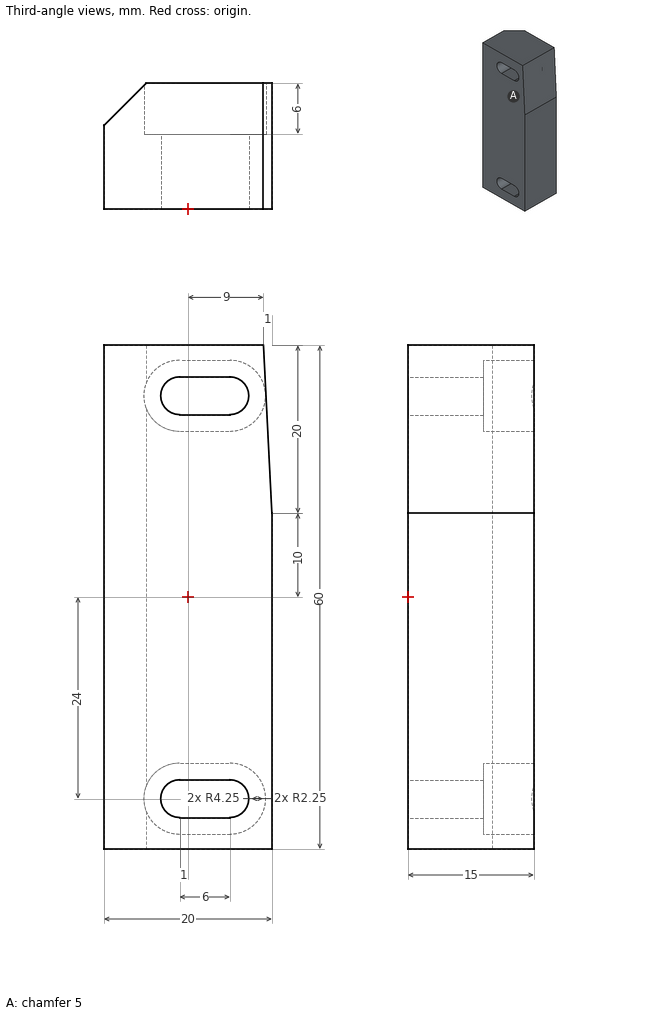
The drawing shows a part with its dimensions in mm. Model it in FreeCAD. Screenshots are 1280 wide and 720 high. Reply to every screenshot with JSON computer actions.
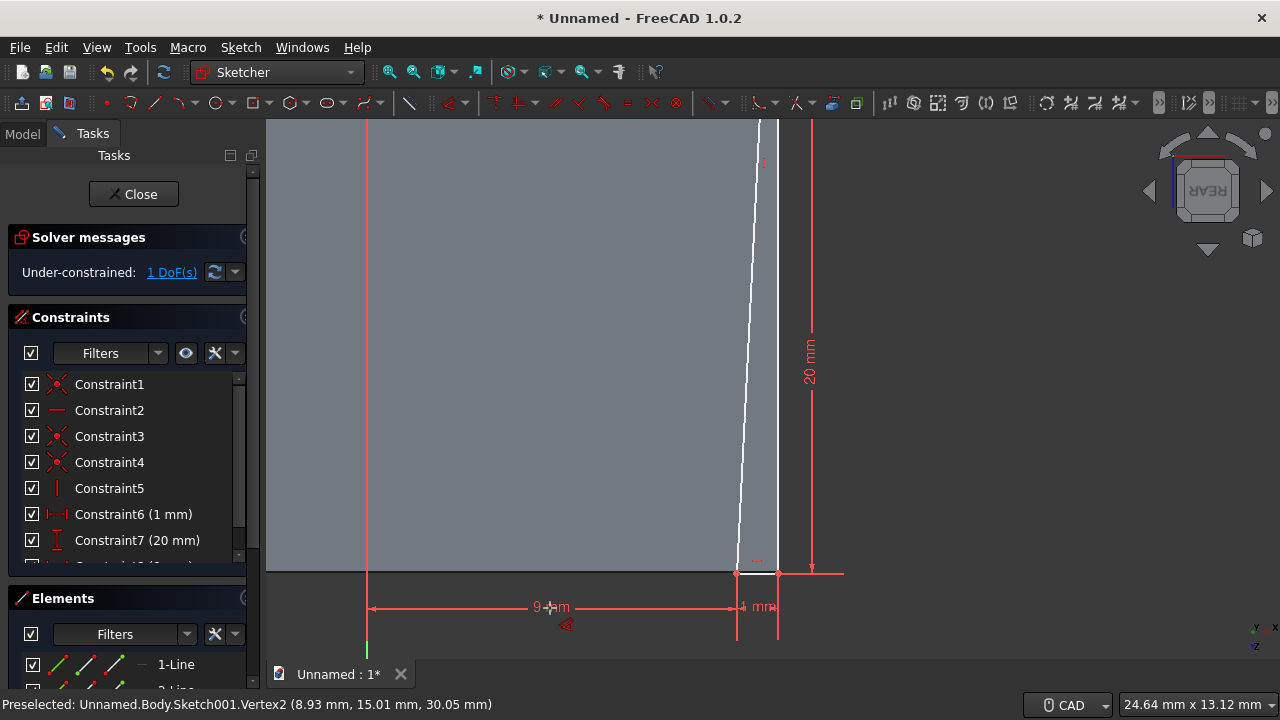
{"action": "scroll", "coordinate": [761, 576], "scroll_direction": "down", "scroll_amount": 6}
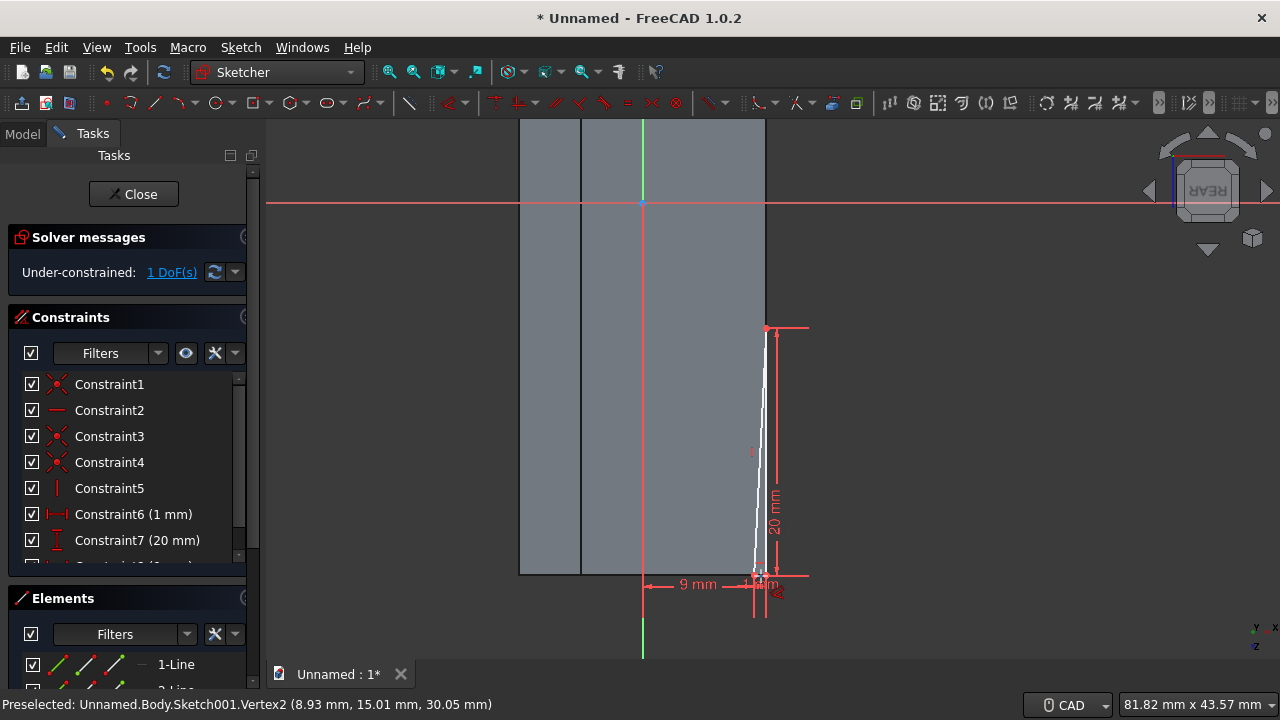
{"action": "left_click", "coordinate": [766, 328]}
{"action": "left_click", "coordinate": [800, 266]}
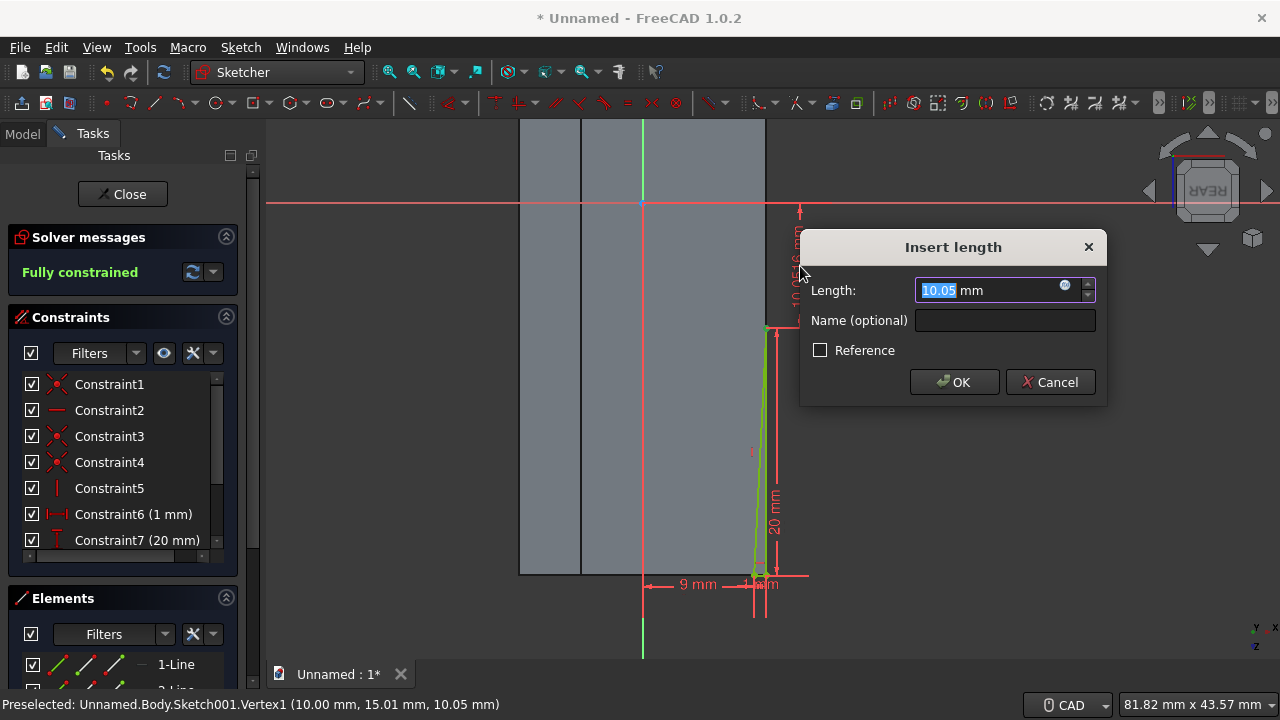
{"action": "type", "text": "10"}
{"action": "key", "text": "Return"}
{"action": "key", "text": "Escape"}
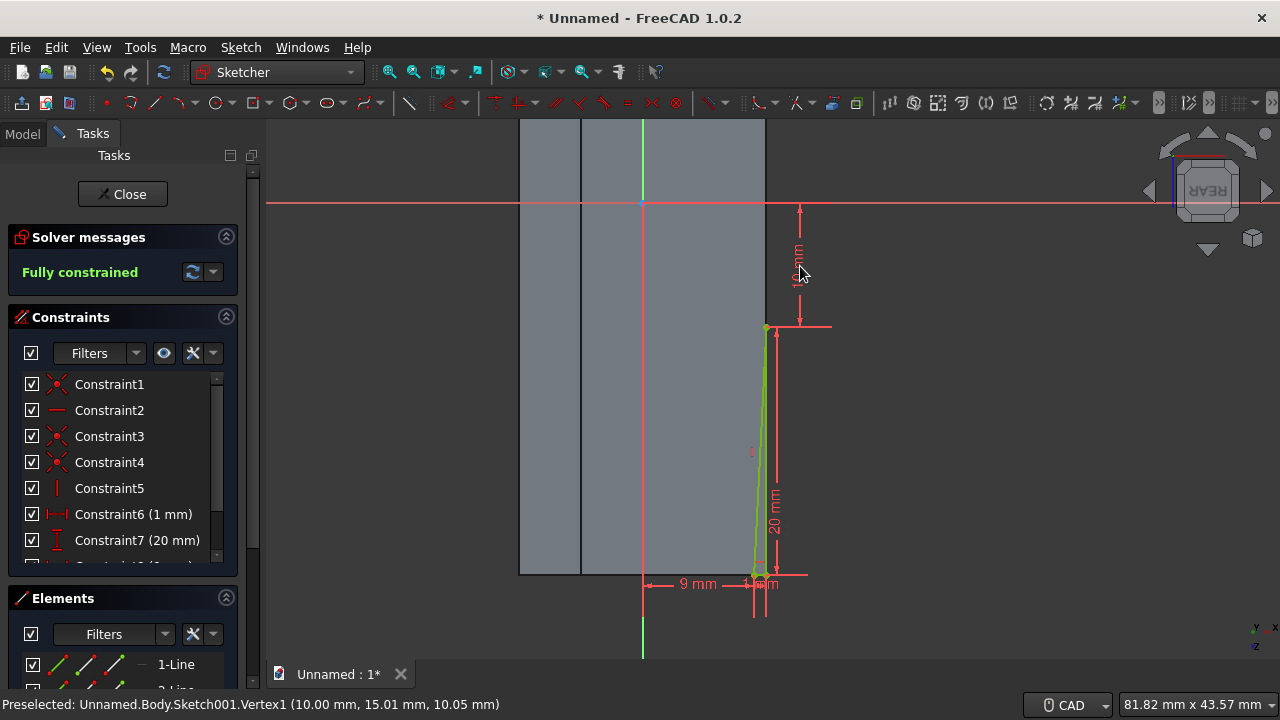
{"action": "left_click", "coordinate": [123, 194]}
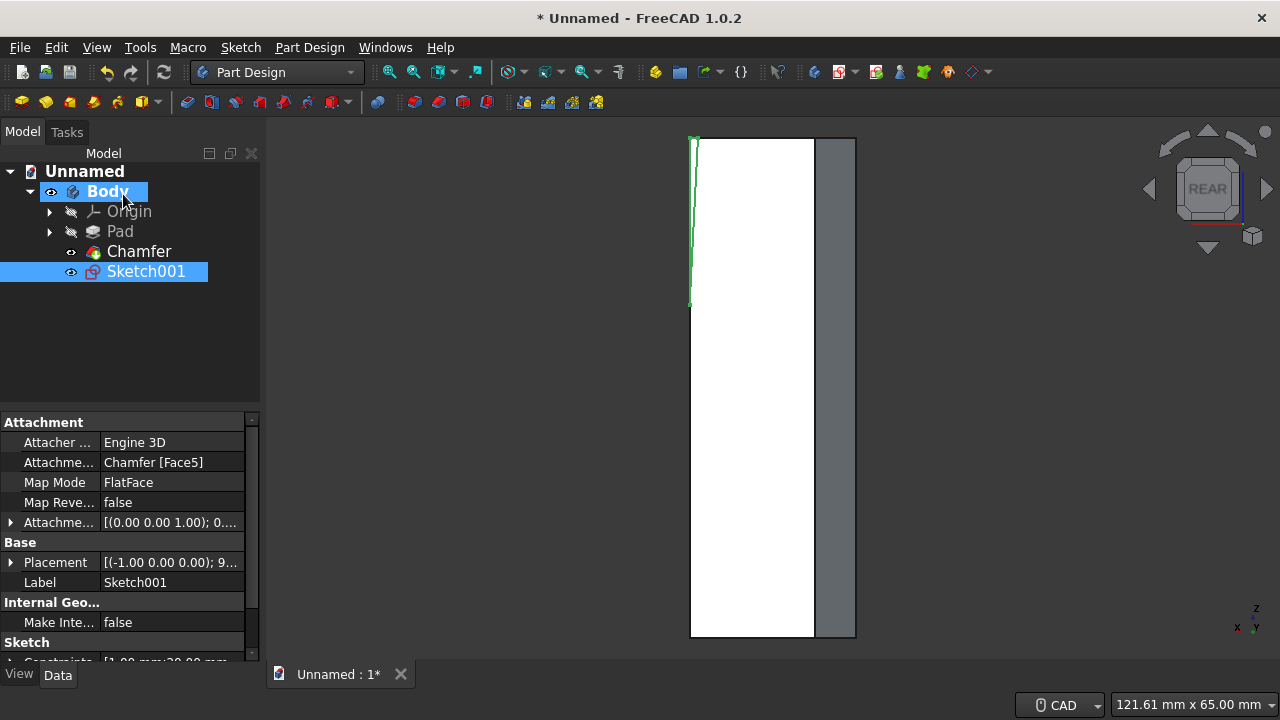
{"action": "left_click", "coordinate": [188, 102]}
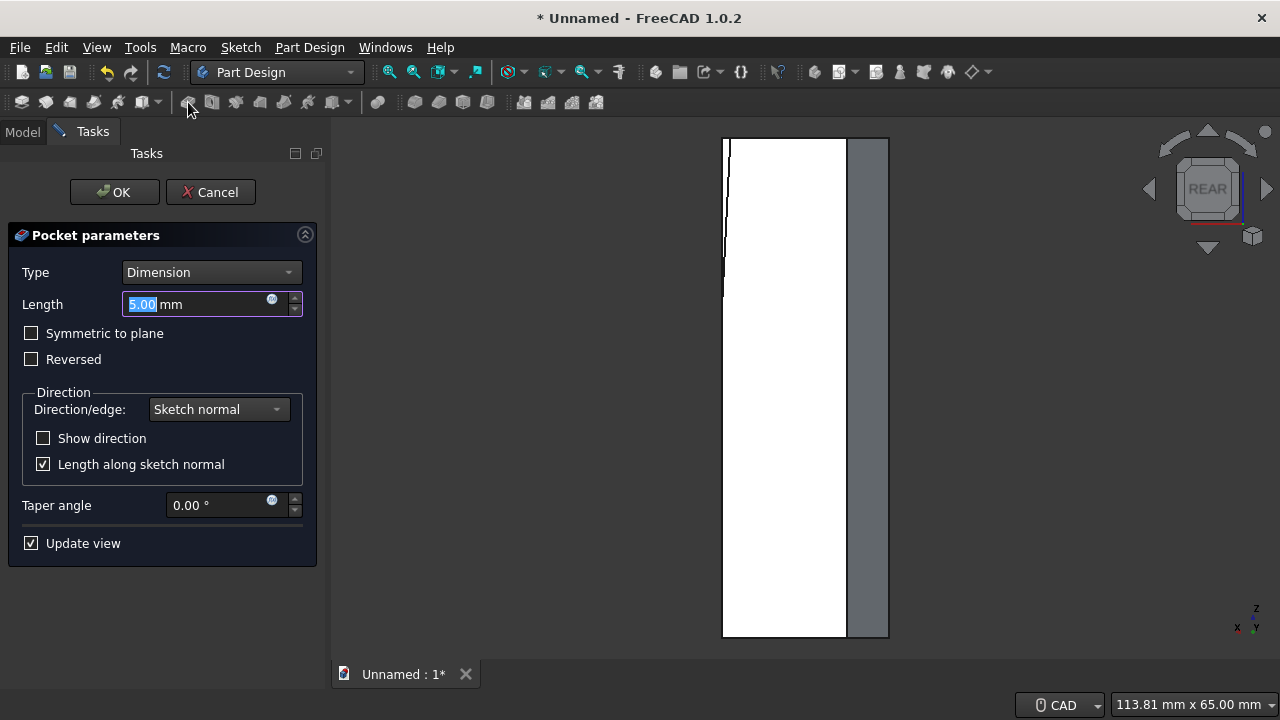
{"action": "left_click", "coordinate": [212, 272]}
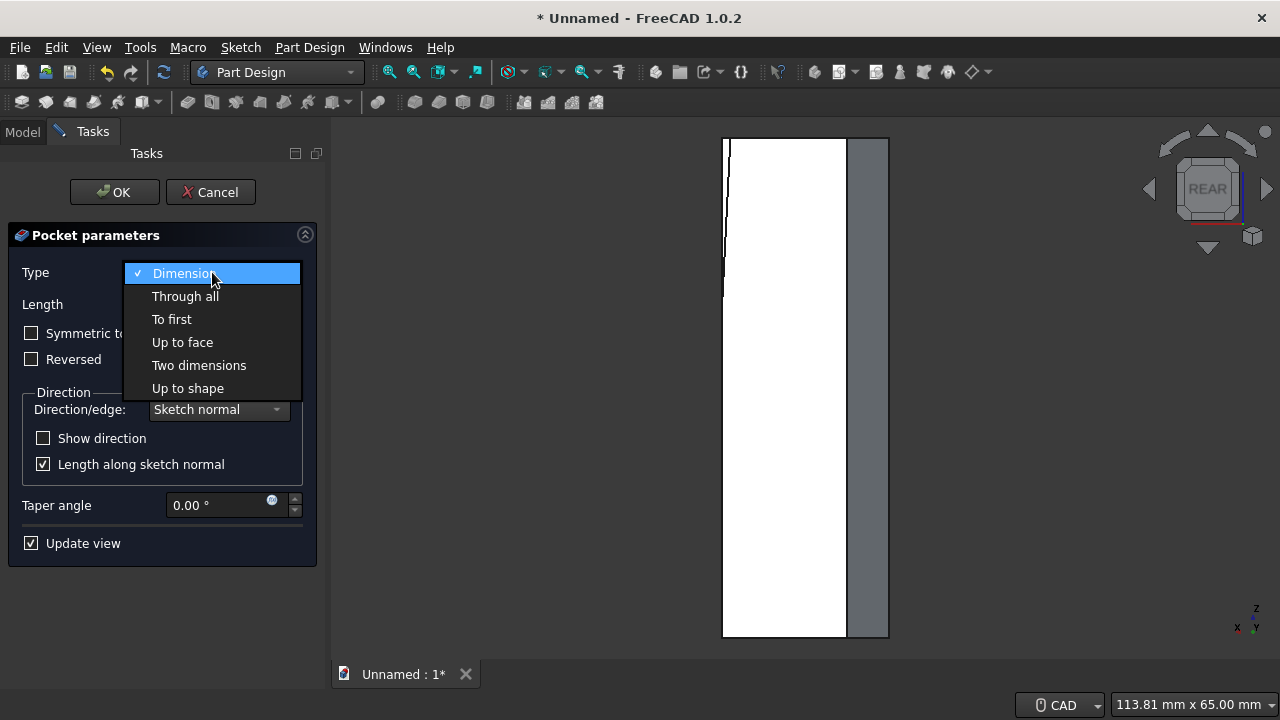
{"action": "left_click", "coordinate": [212, 296]}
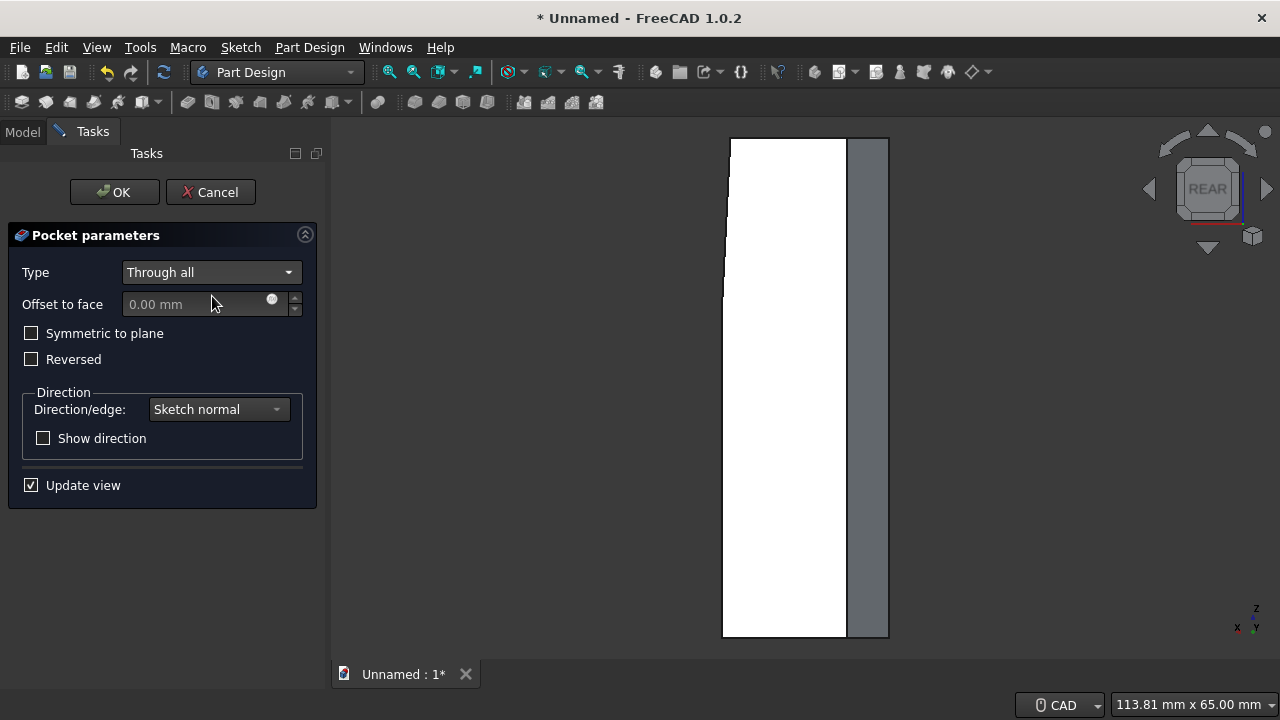
{"action": "left_click", "coordinate": [115, 192]}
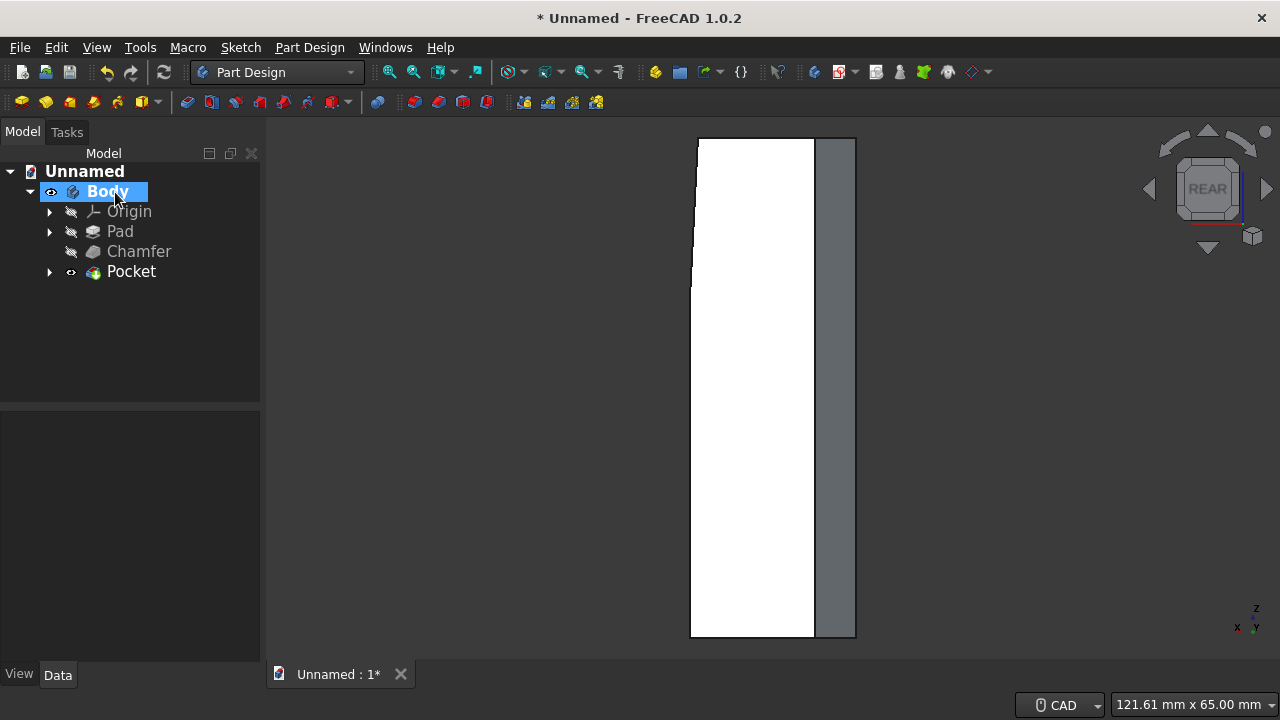
{"action": "left_click", "coordinate": [752, 316]}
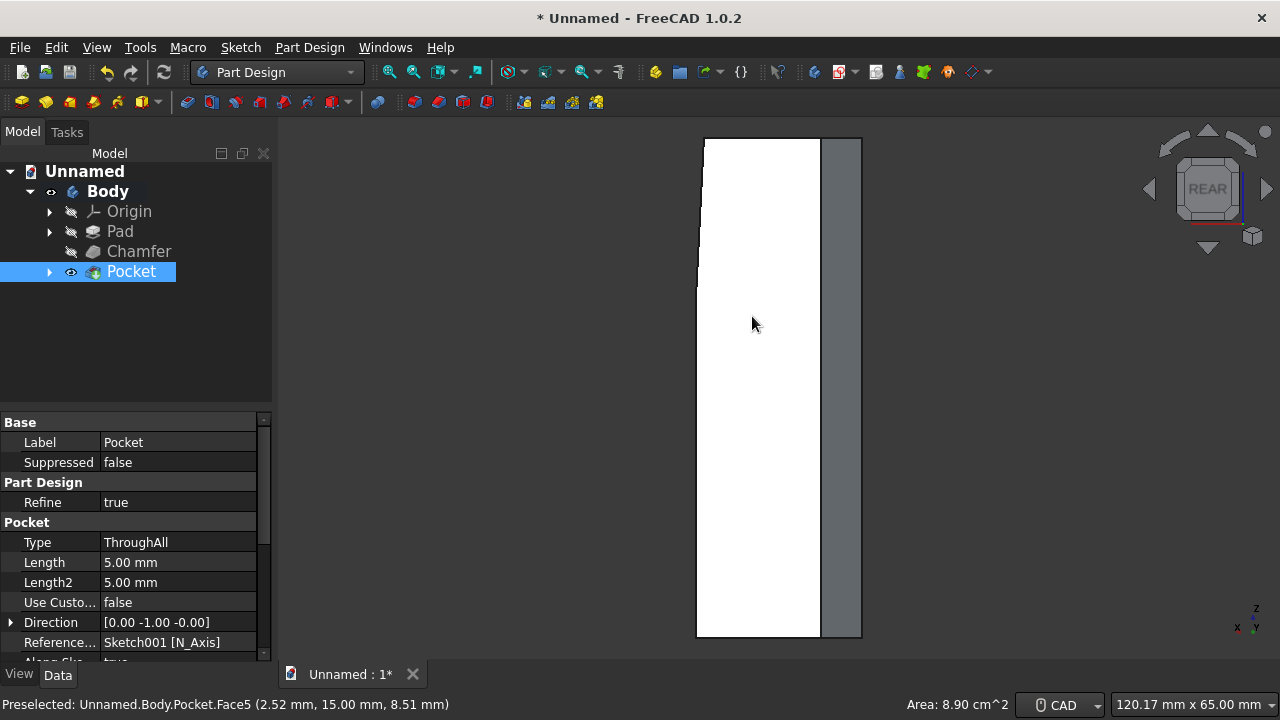
{"action": "left_click", "coordinate": [840, 72]}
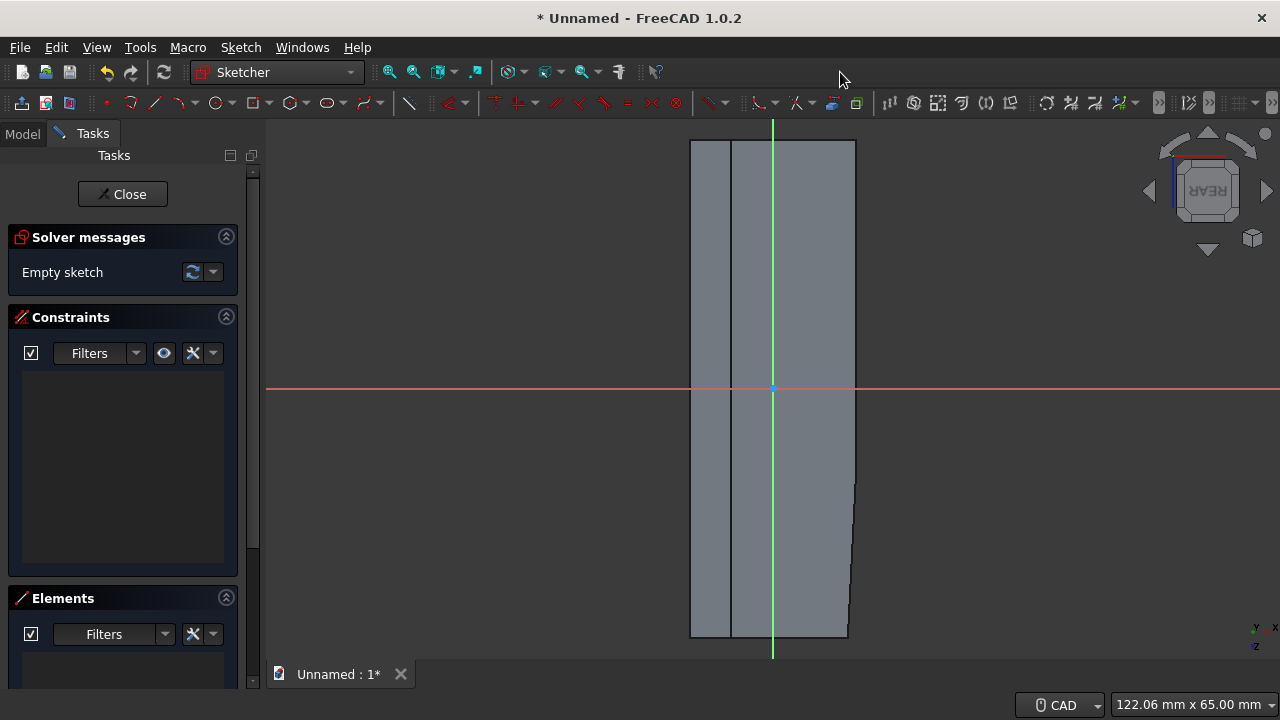
{"action": "scroll", "coordinate": [806, 150], "scroll_direction": "up", "scroll_amount": 9}